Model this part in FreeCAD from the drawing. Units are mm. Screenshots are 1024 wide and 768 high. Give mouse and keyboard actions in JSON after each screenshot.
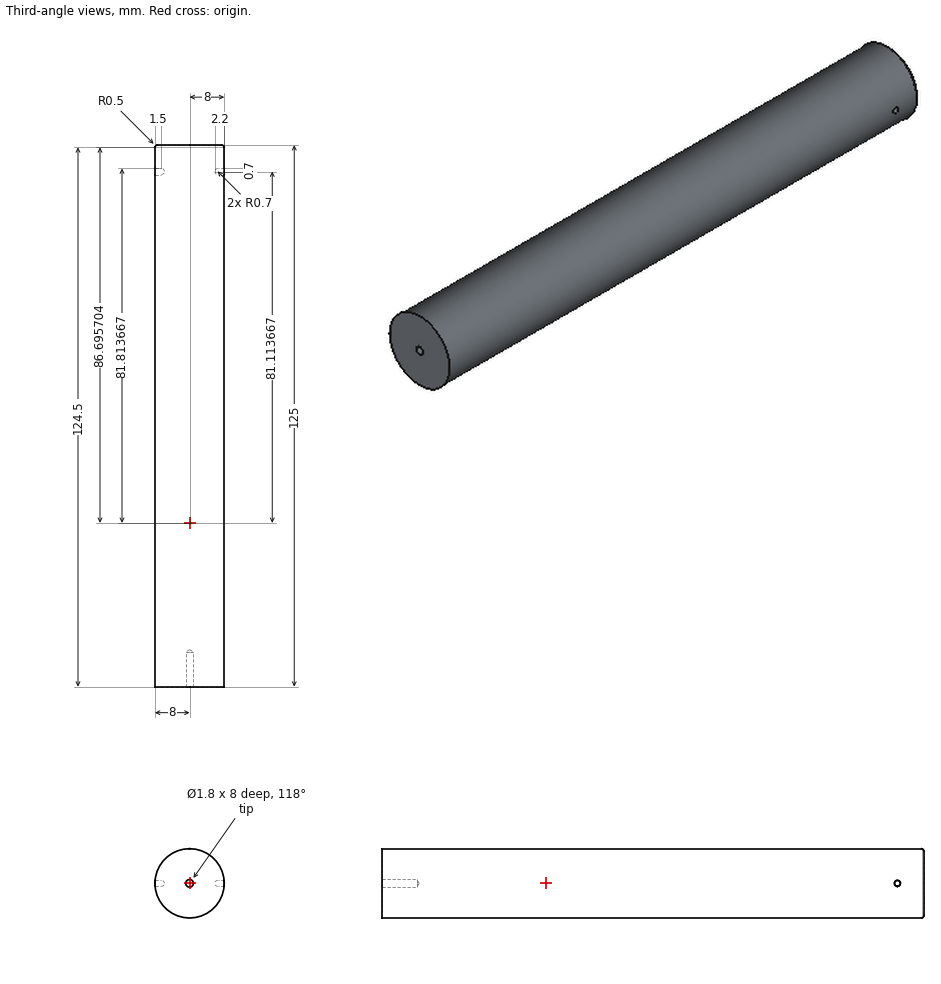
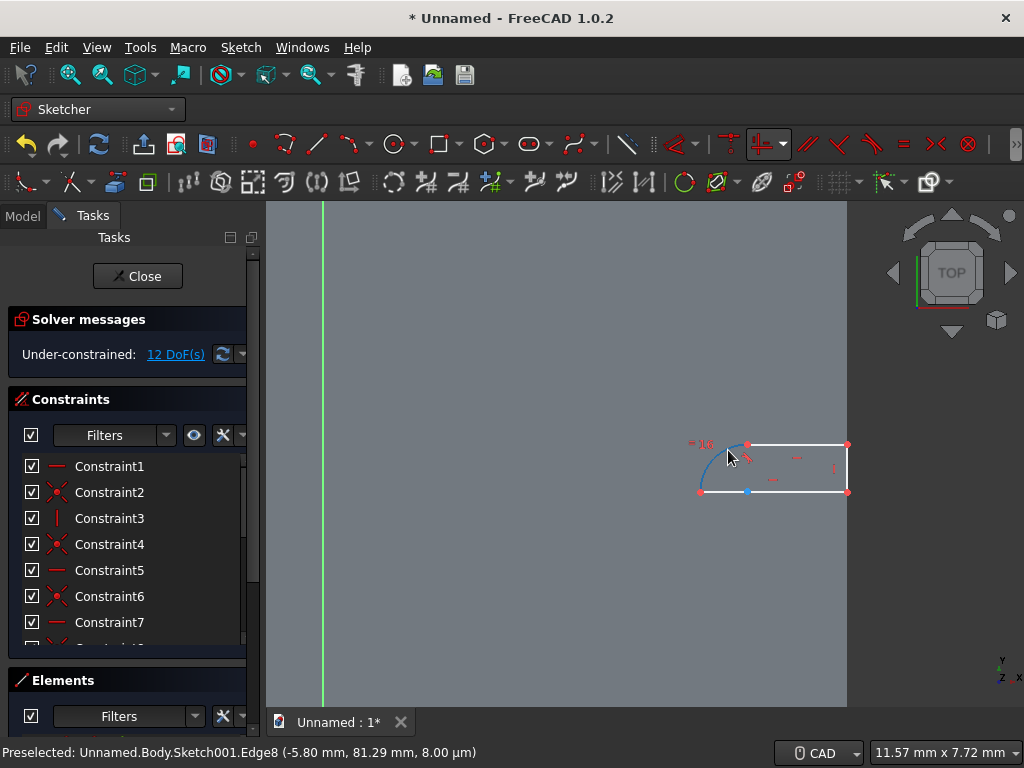
{"action": "left_click", "coordinate": [726, 450]}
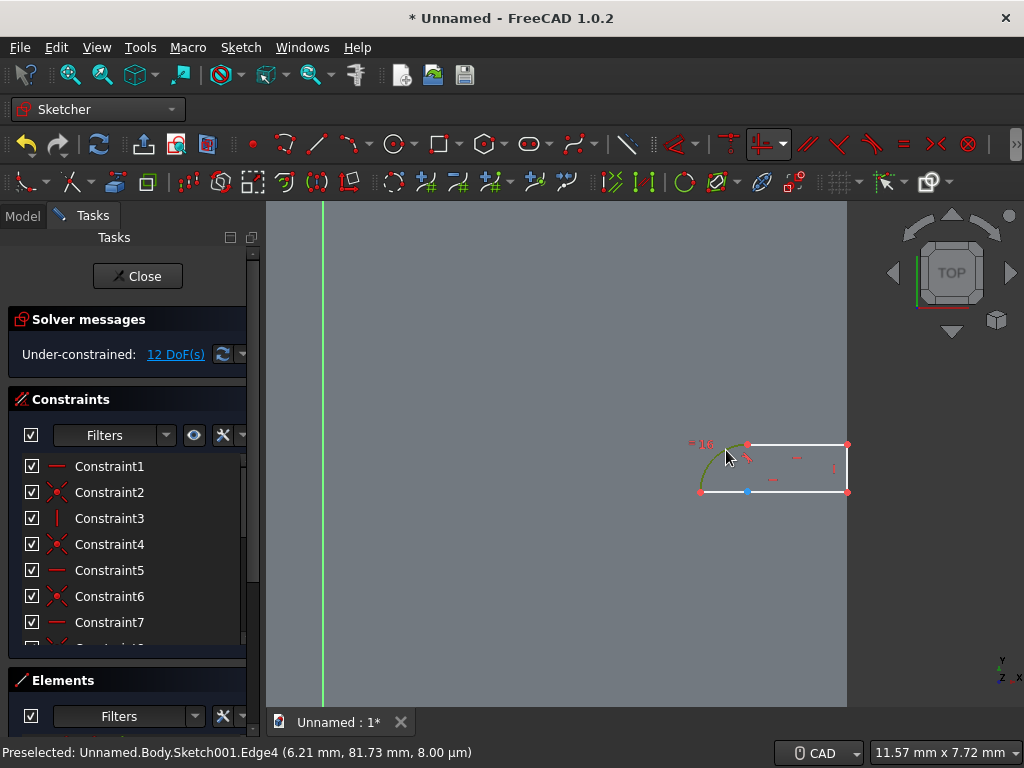
{"action": "left_click", "coordinate": [698, 144]}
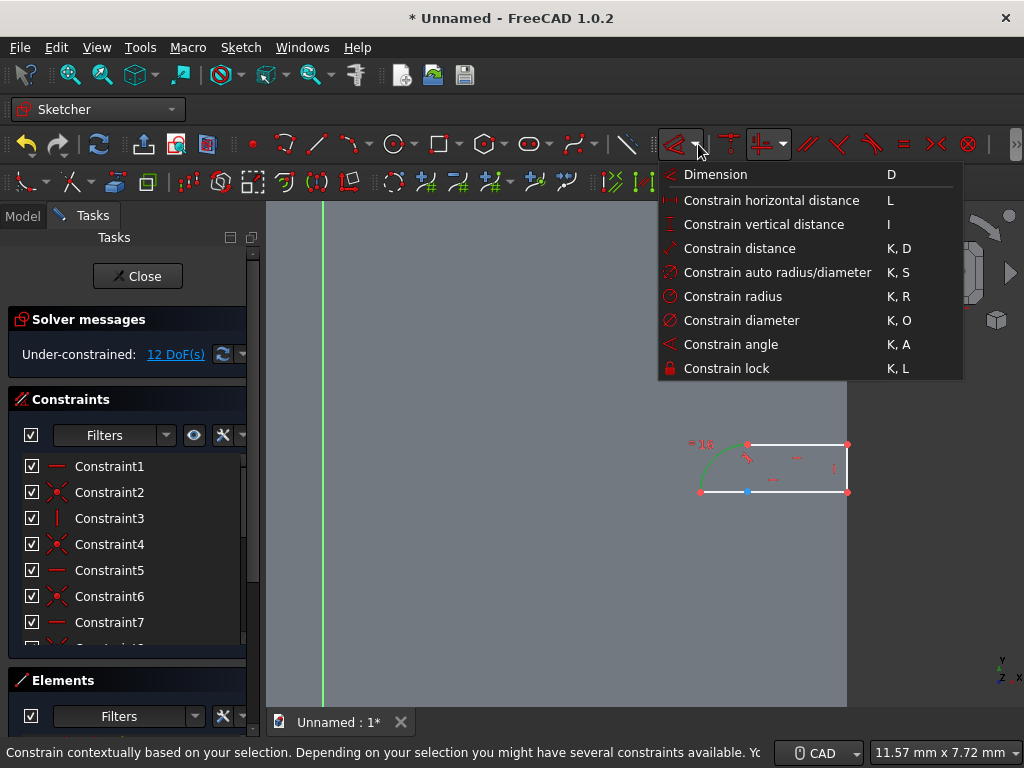
{"action": "left_click", "coordinate": [811, 296]}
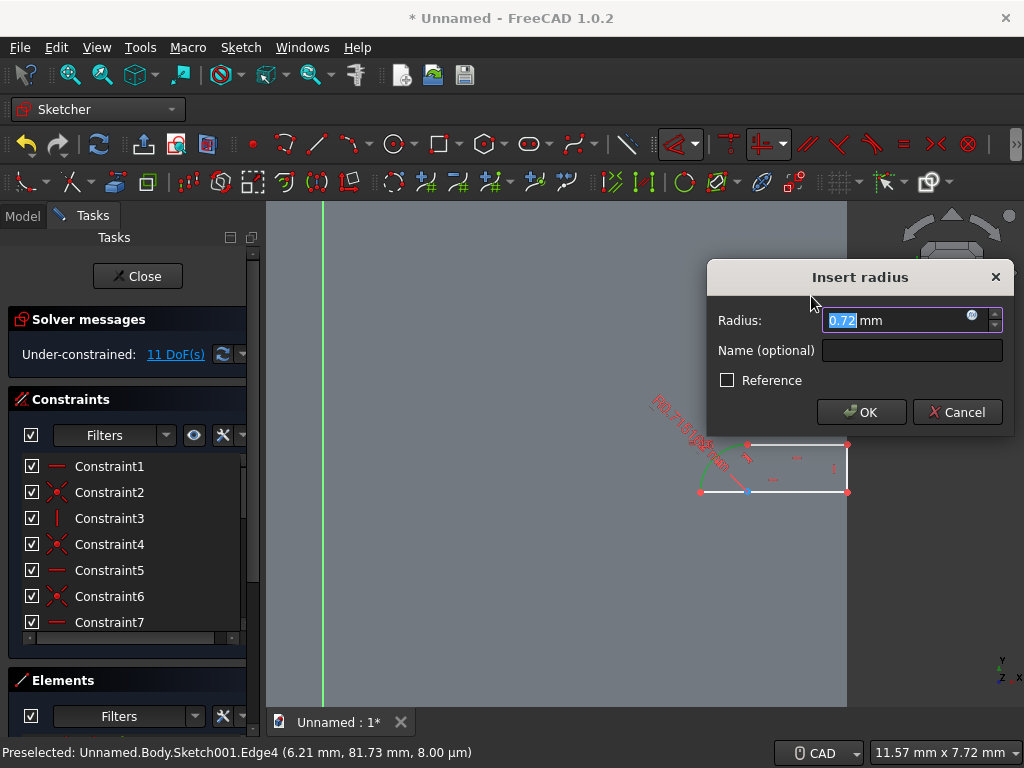
{"action": "type", "text": "0.7"}
{"action": "key", "text": "Return"}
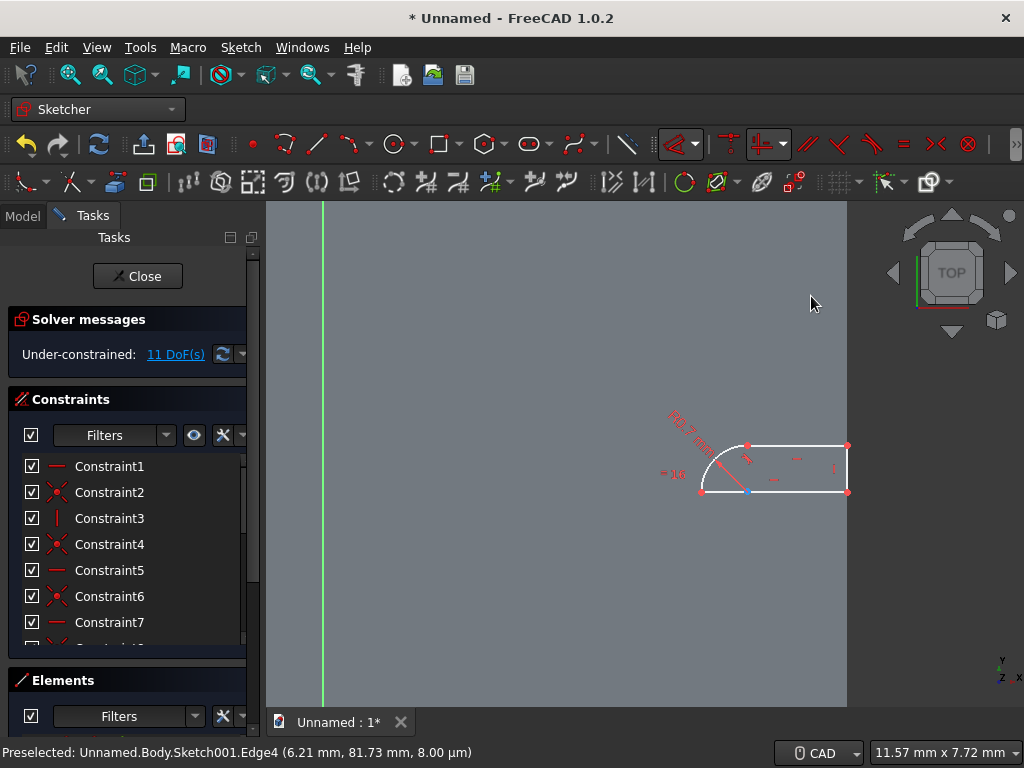
{"action": "scroll", "coordinate": [728, 450], "scroll_direction": "down", "scroll_amount": 7}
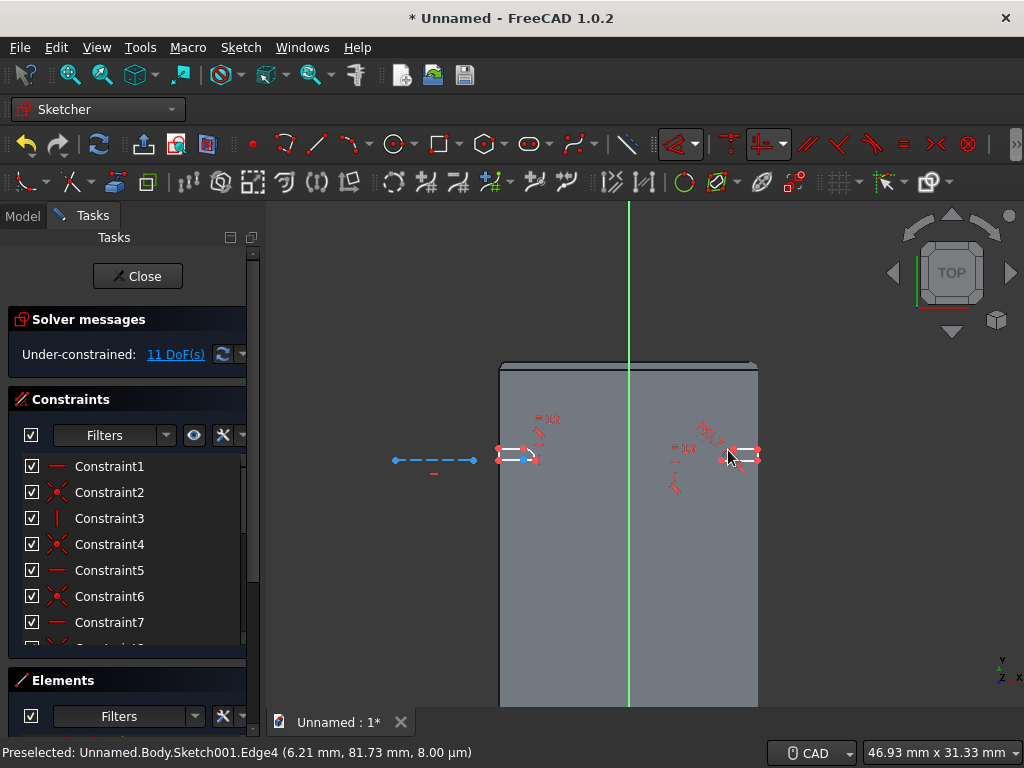
{"action": "left_click", "coordinate": [758, 461]}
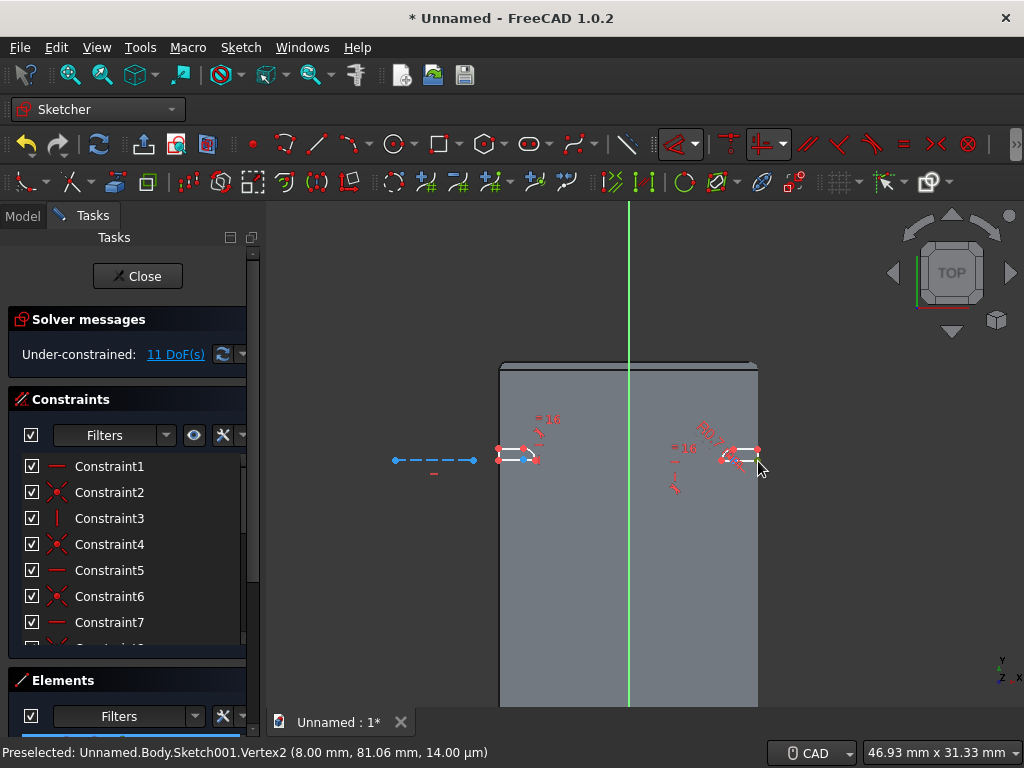
{"action": "left_click", "coordinate": [698, 144]}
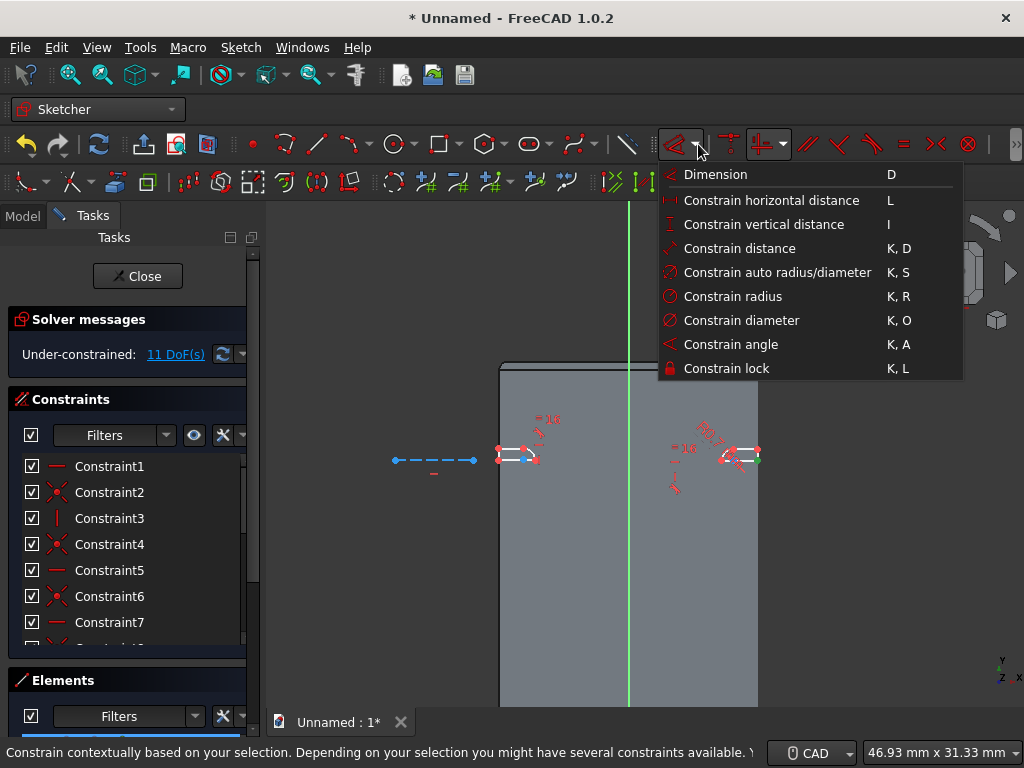
{"action": "left_click", "coordinate": [811, 200]}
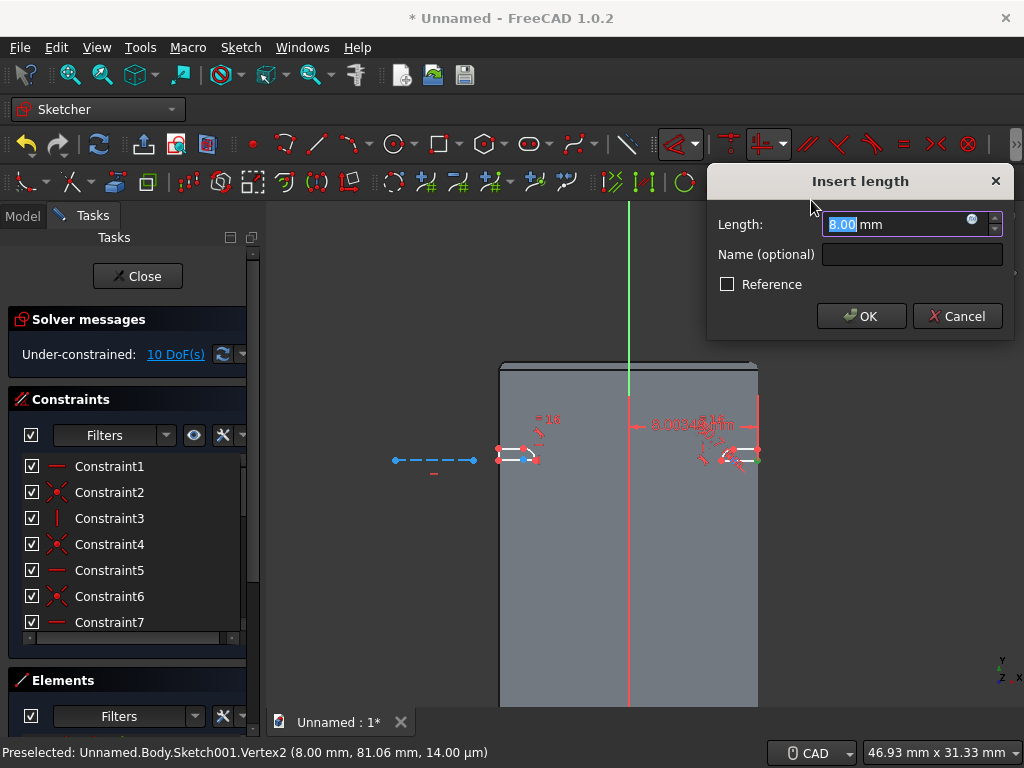
{"action": "type", "text": "8"}
{"action": "key", "text": "Return"}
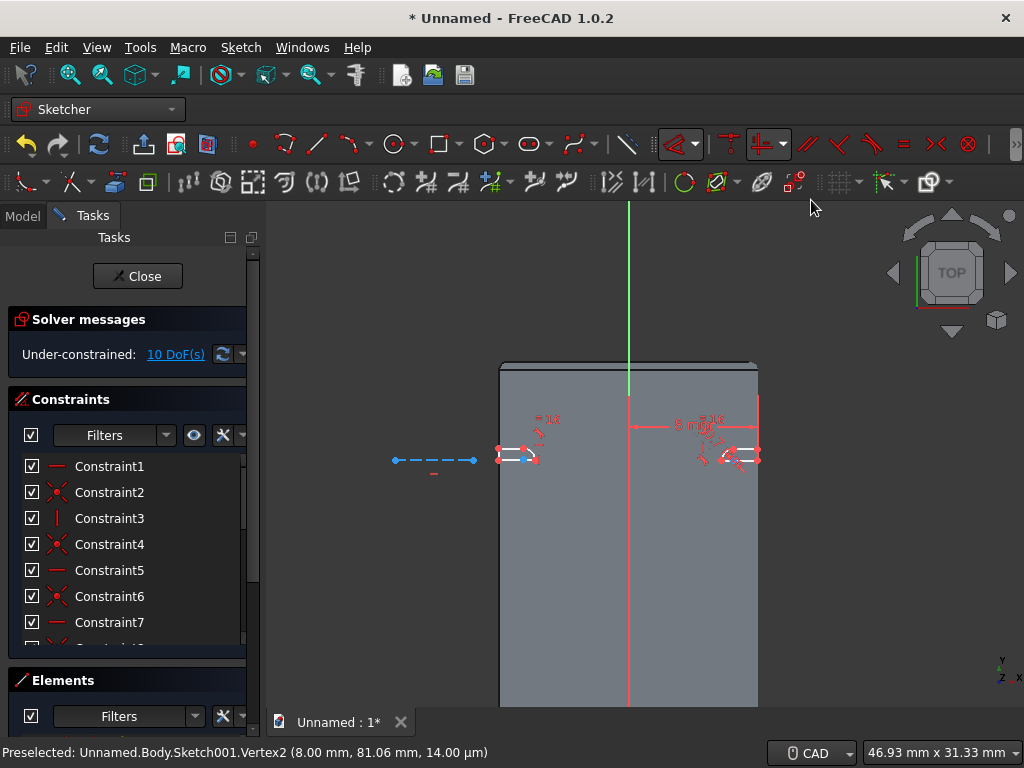
{"action": "left_click", "coordinate": [499, 449]}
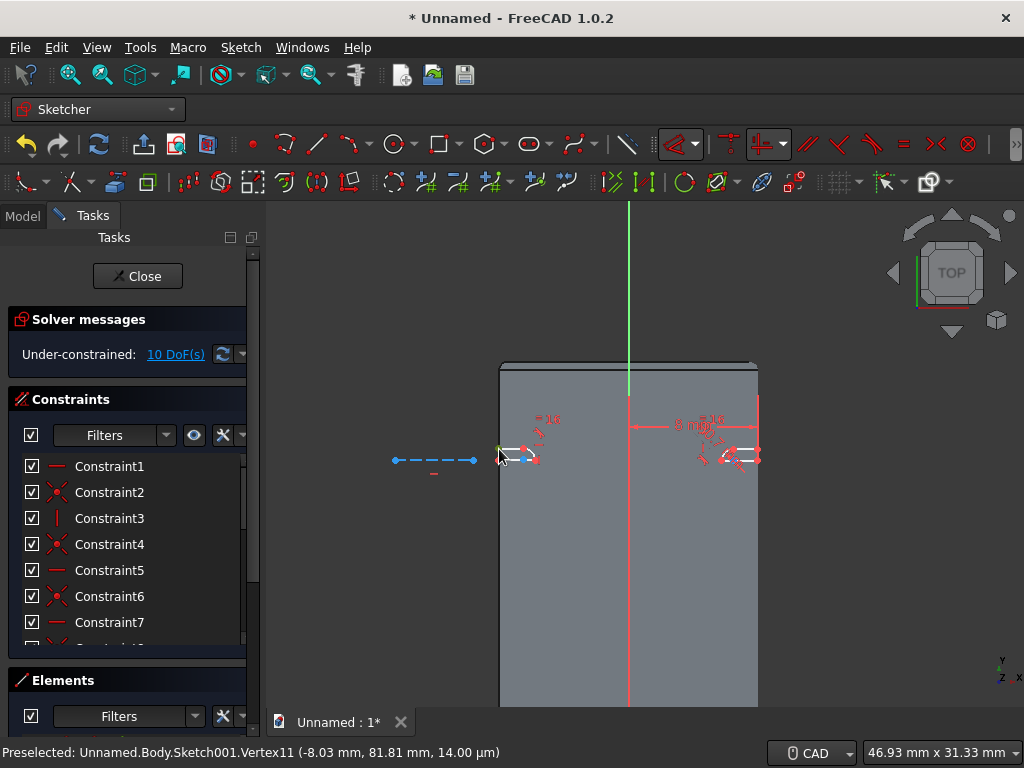
{"action": "key", "text": "l"}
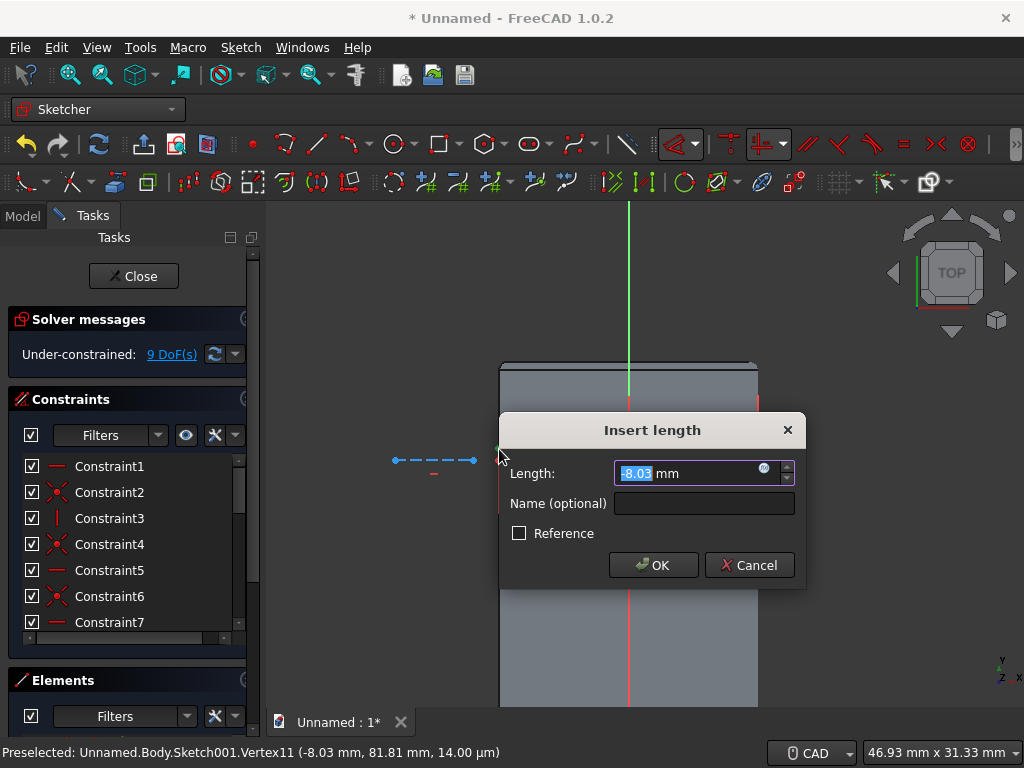
{"action": "type", "text": "-8"}
{"action": "key", "text": "Return"}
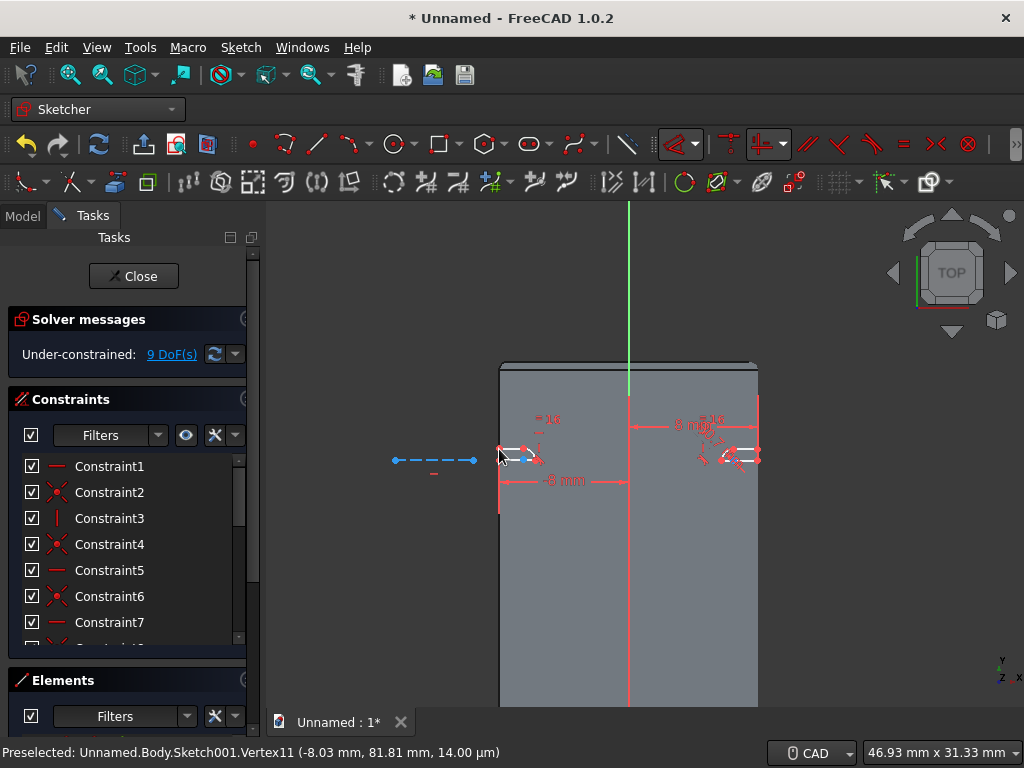
{"action": "scroll", "coordinate": [733, 461], "scroll_direction": "up", "scroll_amount": 2}